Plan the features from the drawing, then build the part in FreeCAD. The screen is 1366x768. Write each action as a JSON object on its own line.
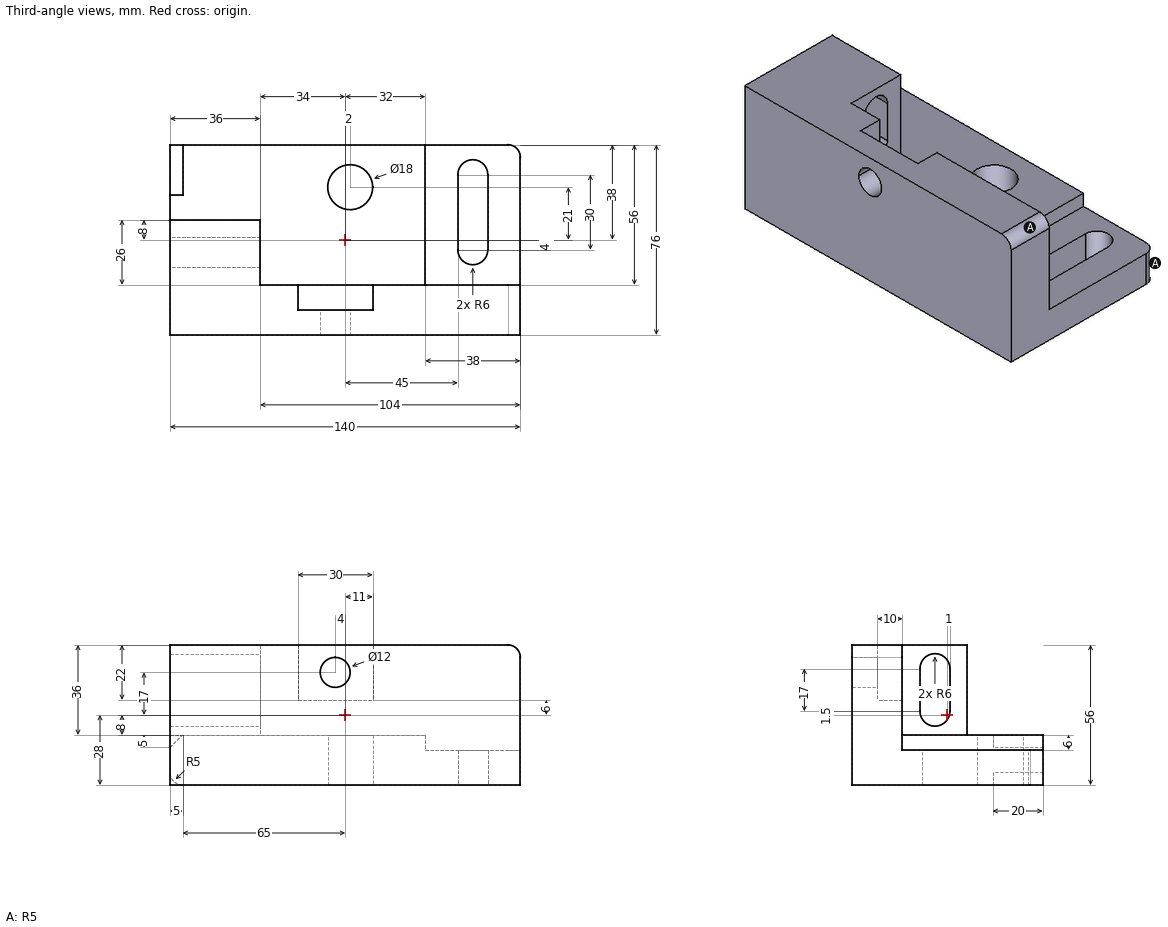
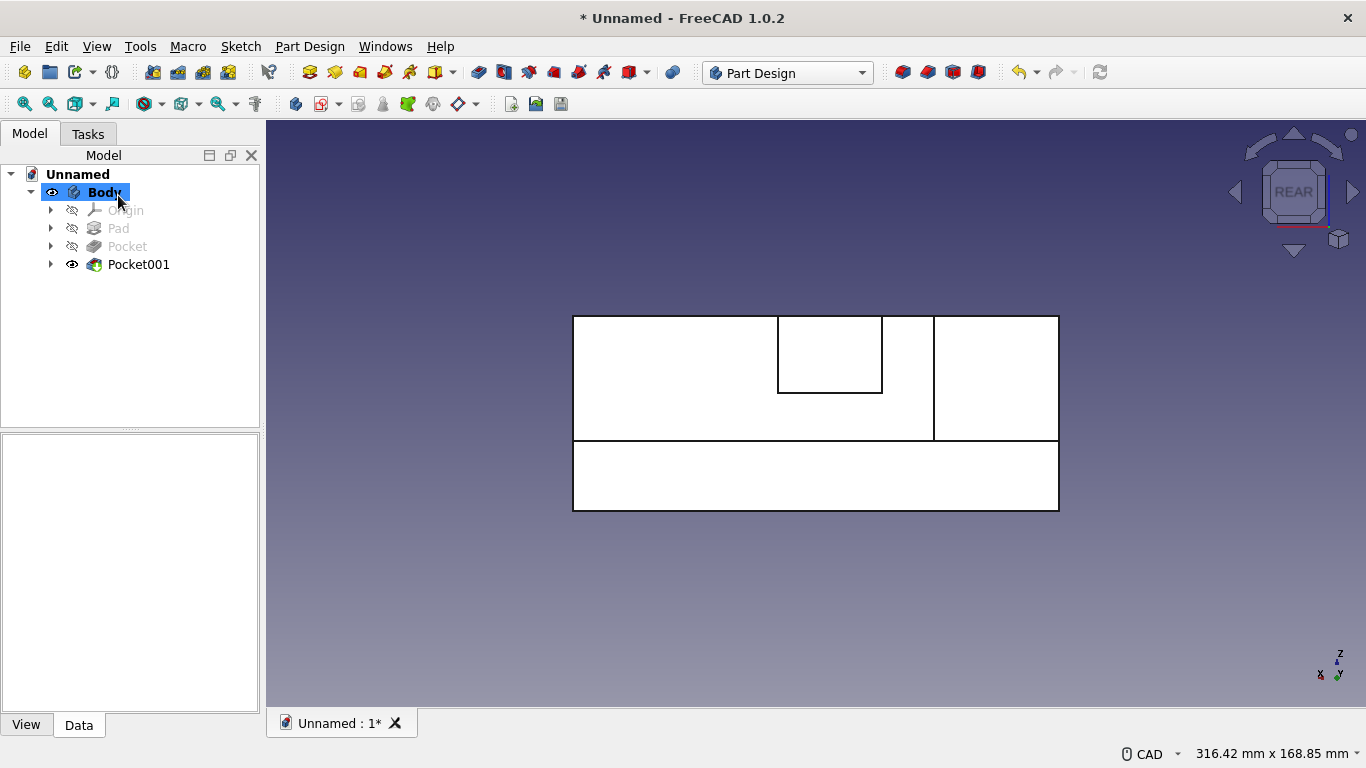
{"action": "left_click", "coordinate": [25, 104]}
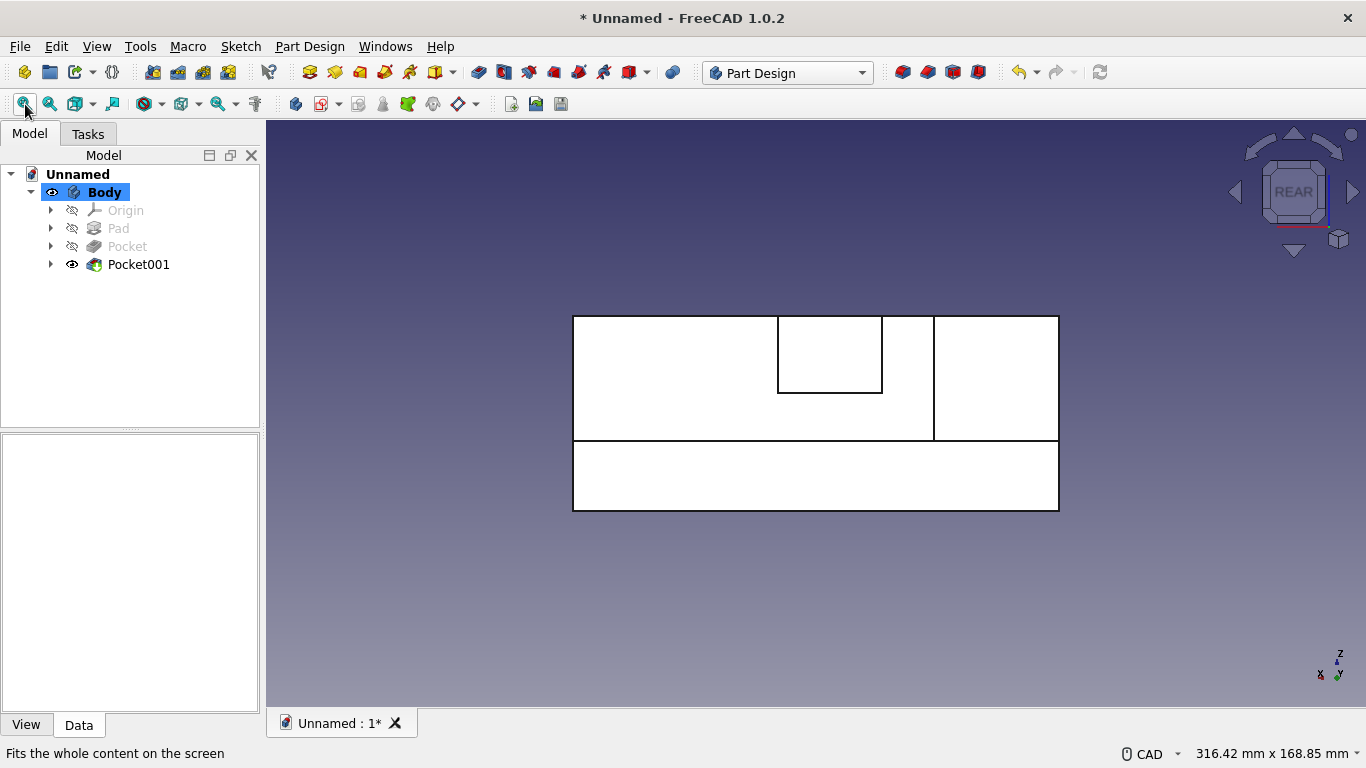
{"action": "key", "text": "0"}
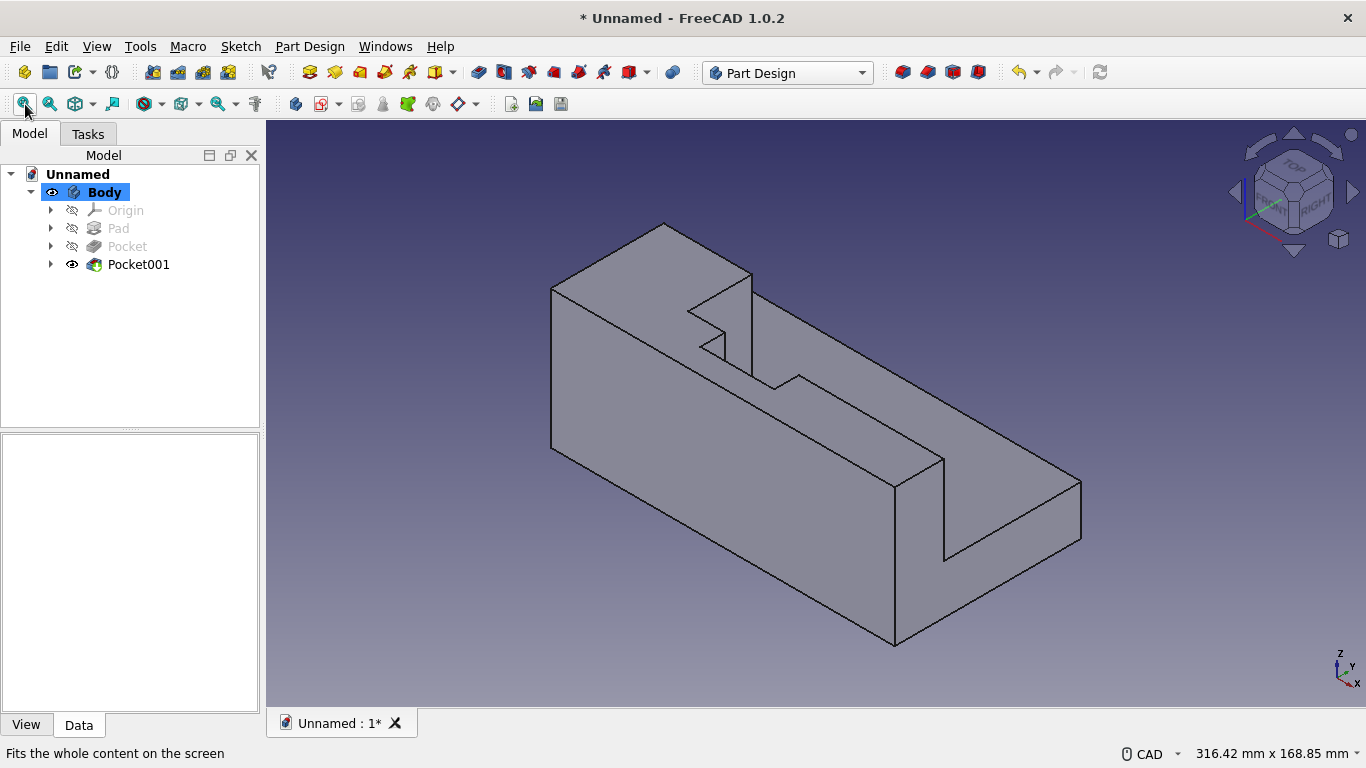
{"action": "left_click", "coordinate": [959, 466]}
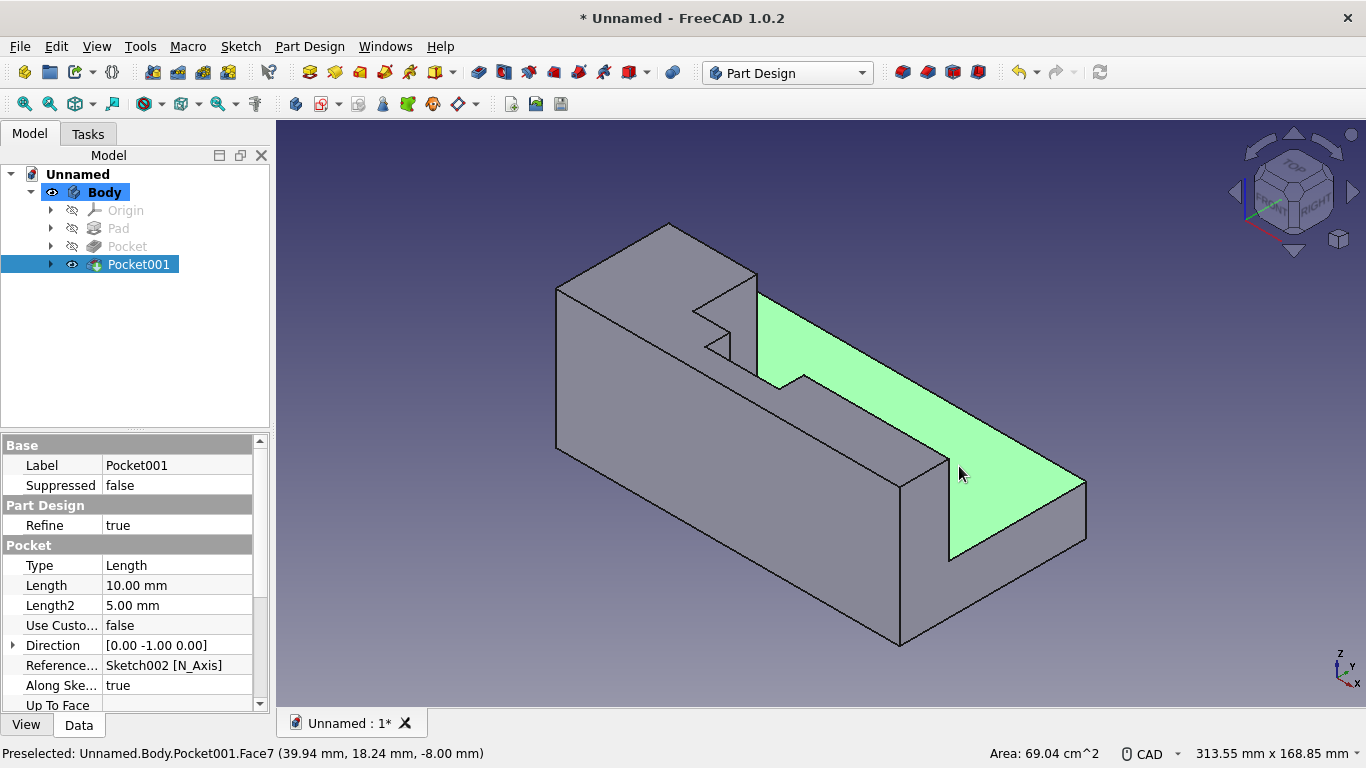
{"action": "left_click", "coordinate": [320, 104]}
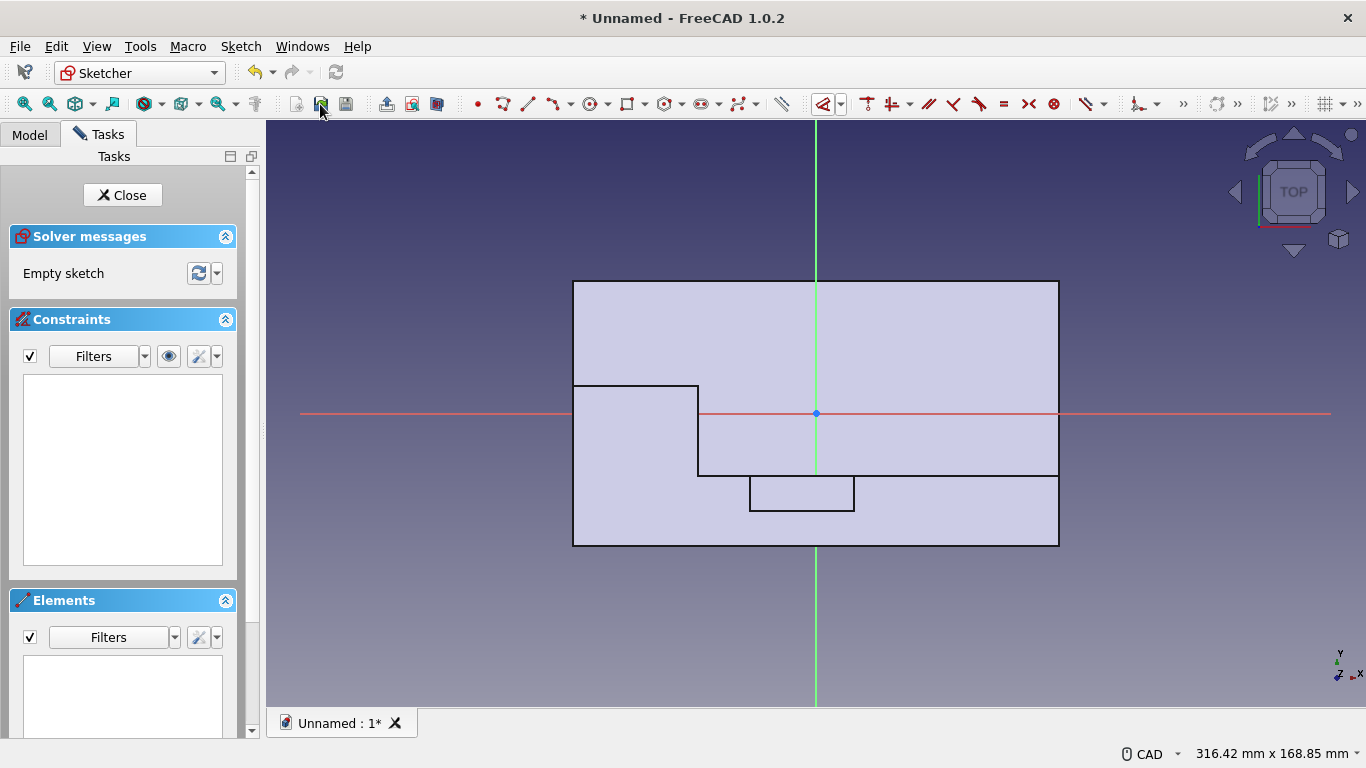
{"action": "left_click", "coordinate": [437, 104]}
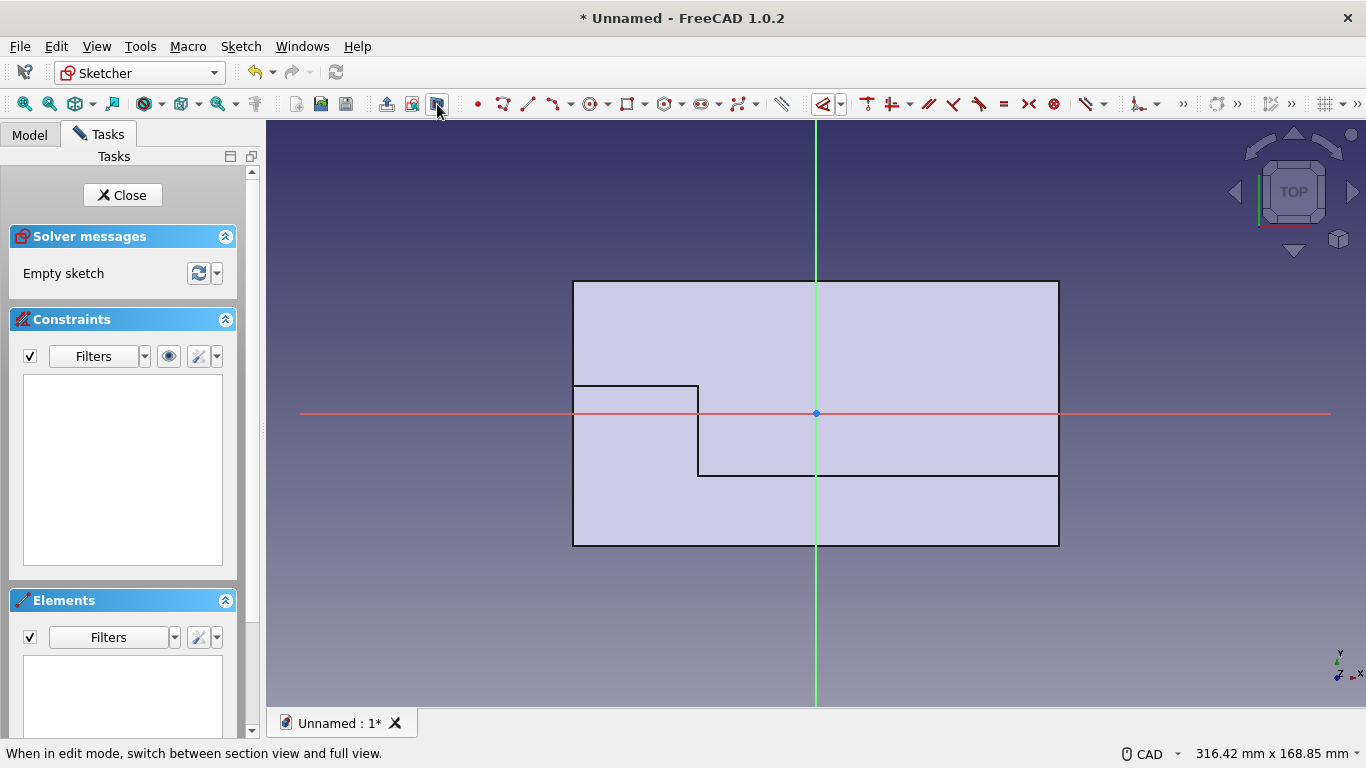
{"action": "scroll", "coordinate": [1169, 336], "scroll_direction": "up", "scroll_amount": 3}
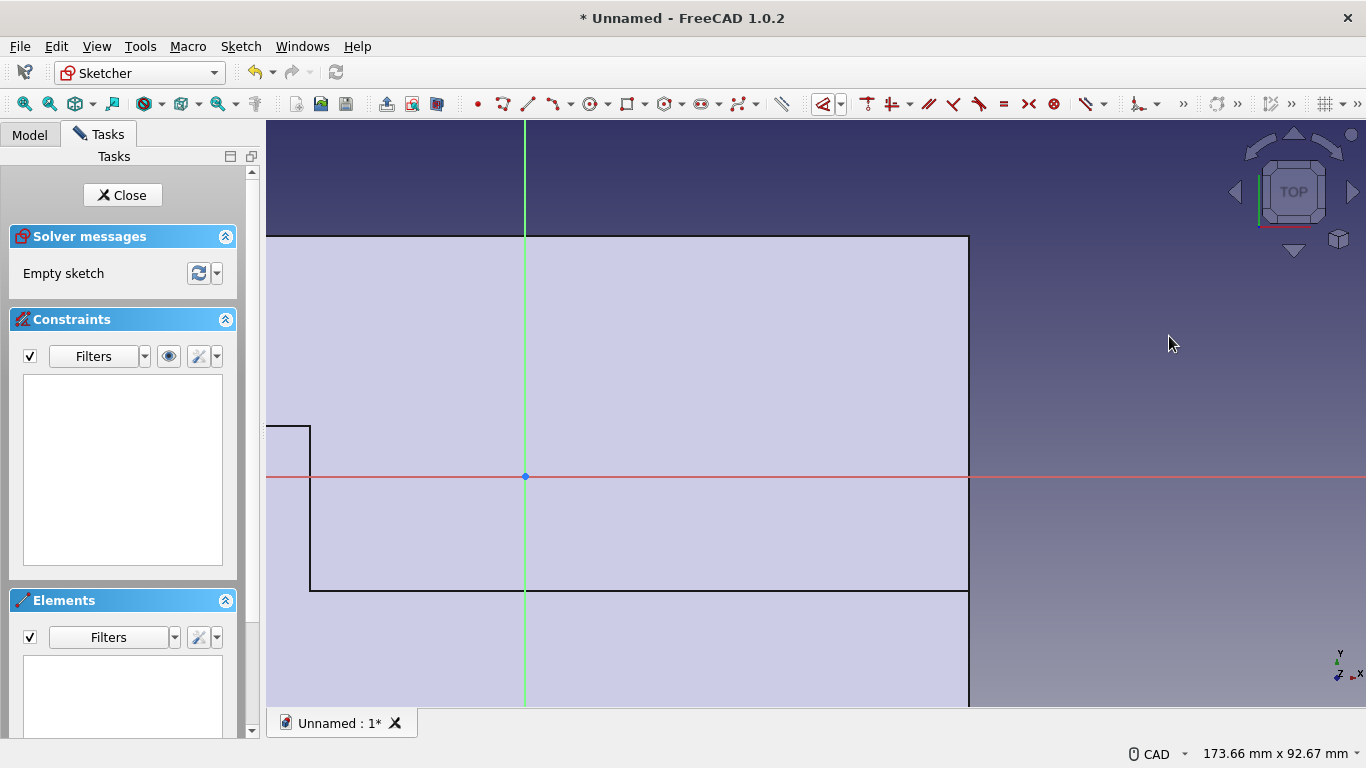
{"action": "left_click", "coordinate": [626, 104]}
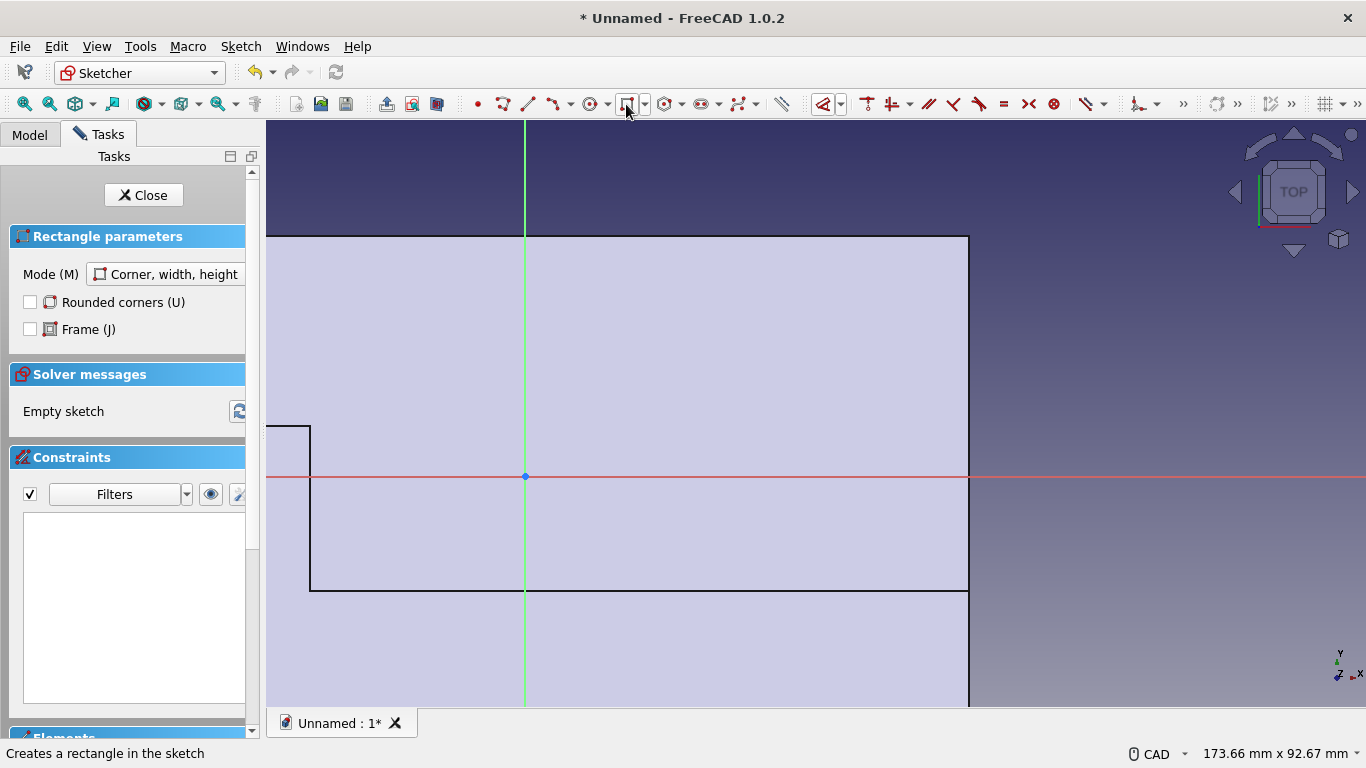
{"action": "left_click", "coordinate": [728, 236]}
{"action": "mouse_move", "coordinate": [969, 591]}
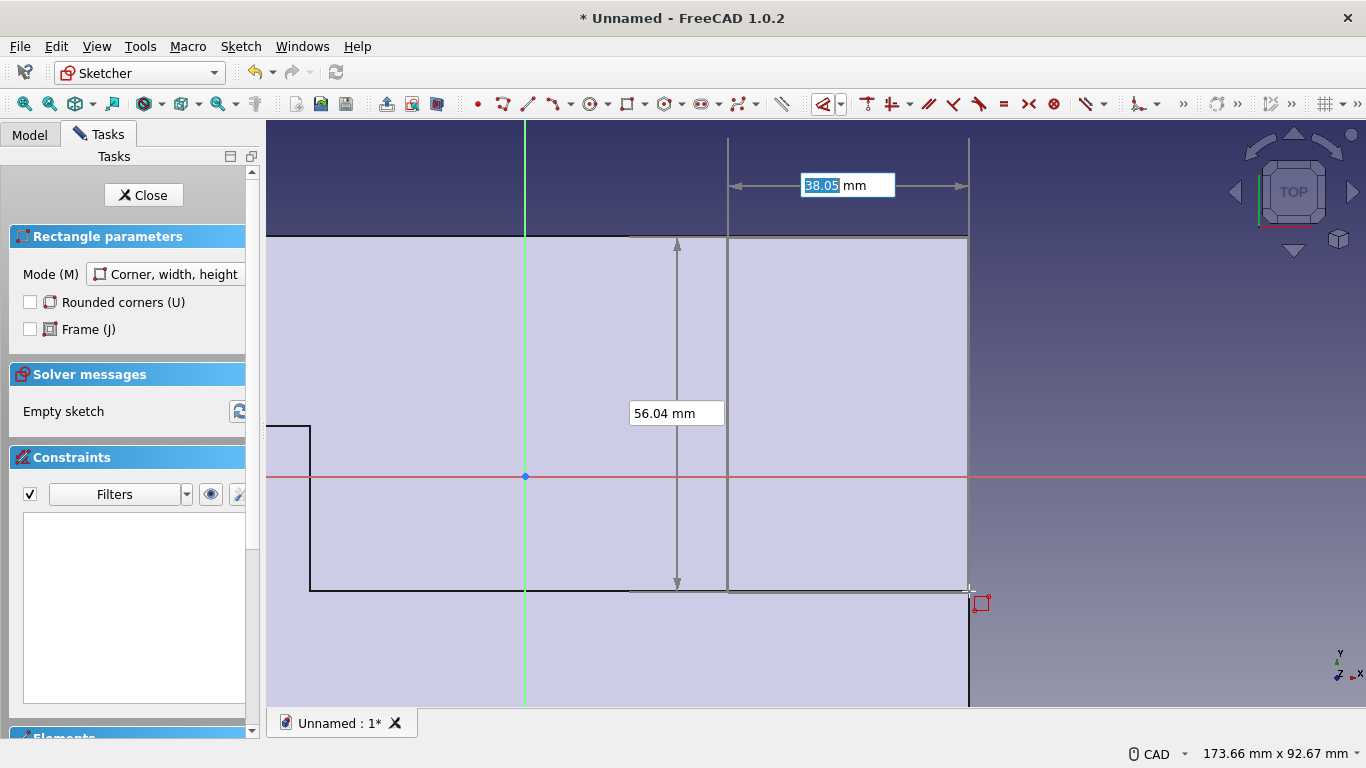
{"action": "type", "text": "38"}
{"action": "key", "text": "Tab"}
{"action": "type", "text": "56"}
{"action": "key", "text": "Return"}
{"action": "key", "text": "Escape"}